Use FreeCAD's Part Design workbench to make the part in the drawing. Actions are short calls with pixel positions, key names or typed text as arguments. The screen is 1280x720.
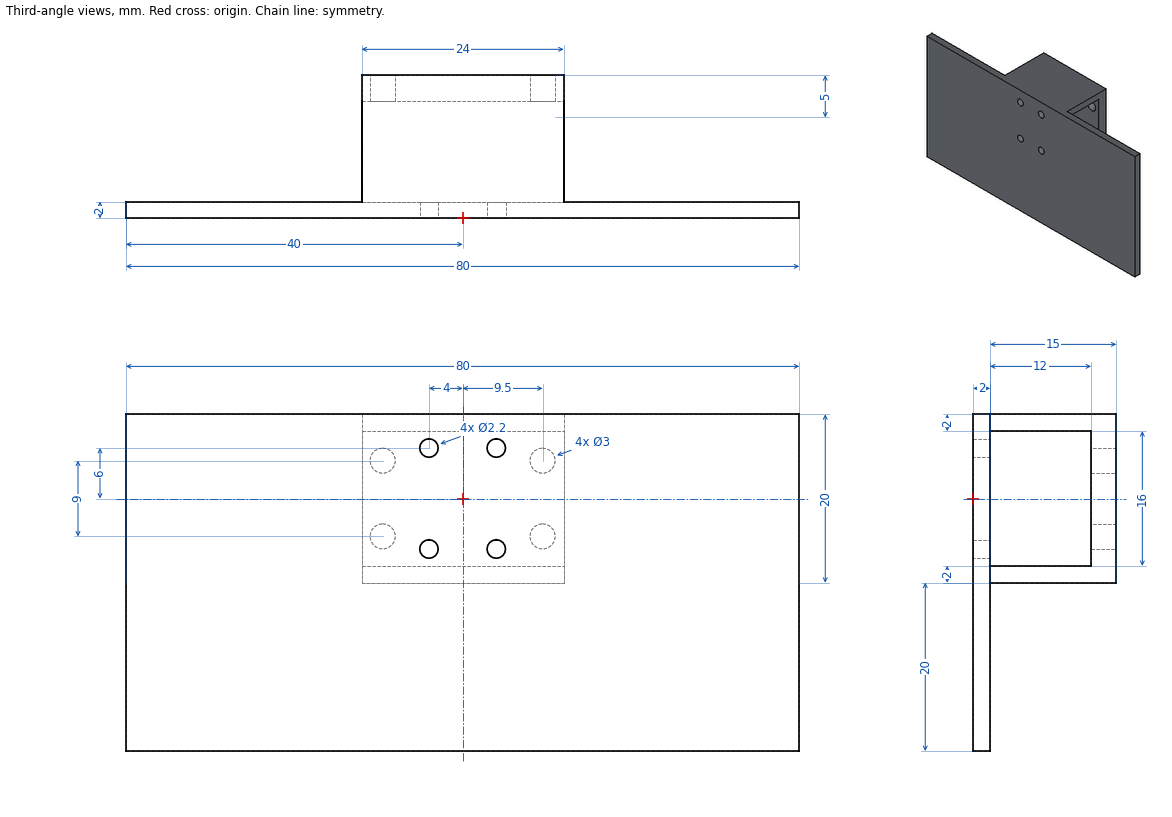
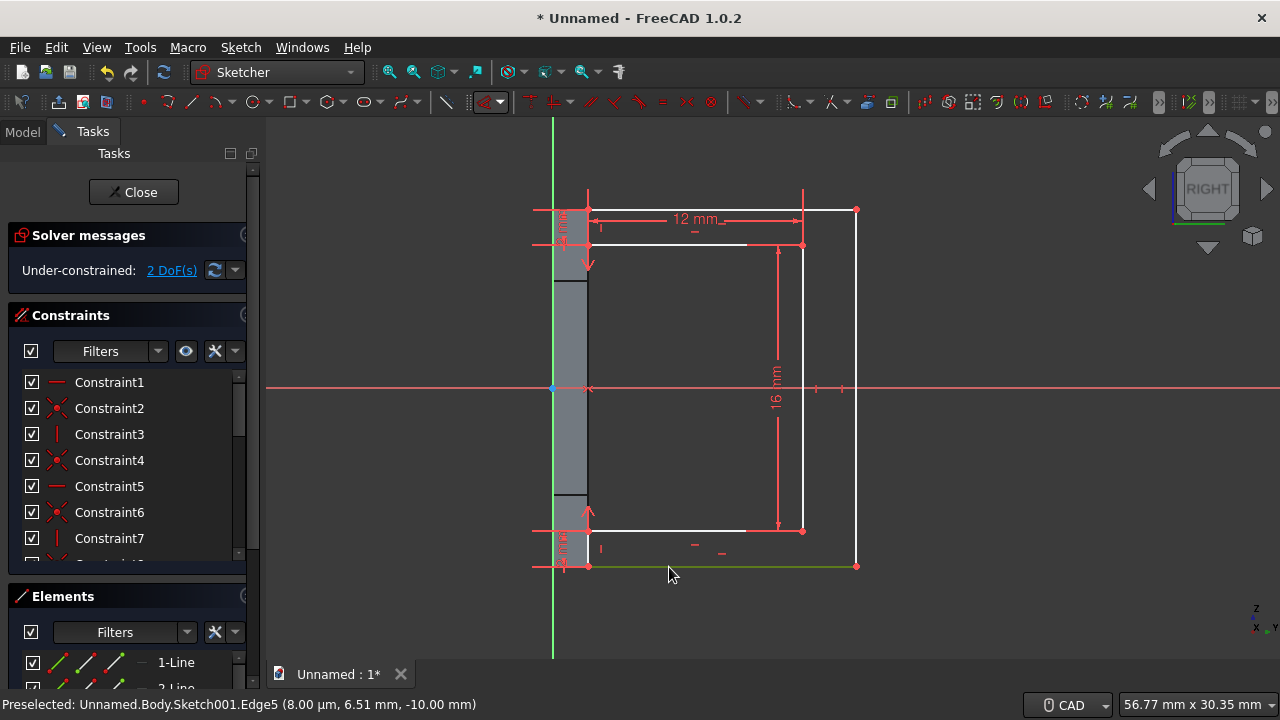
key(l)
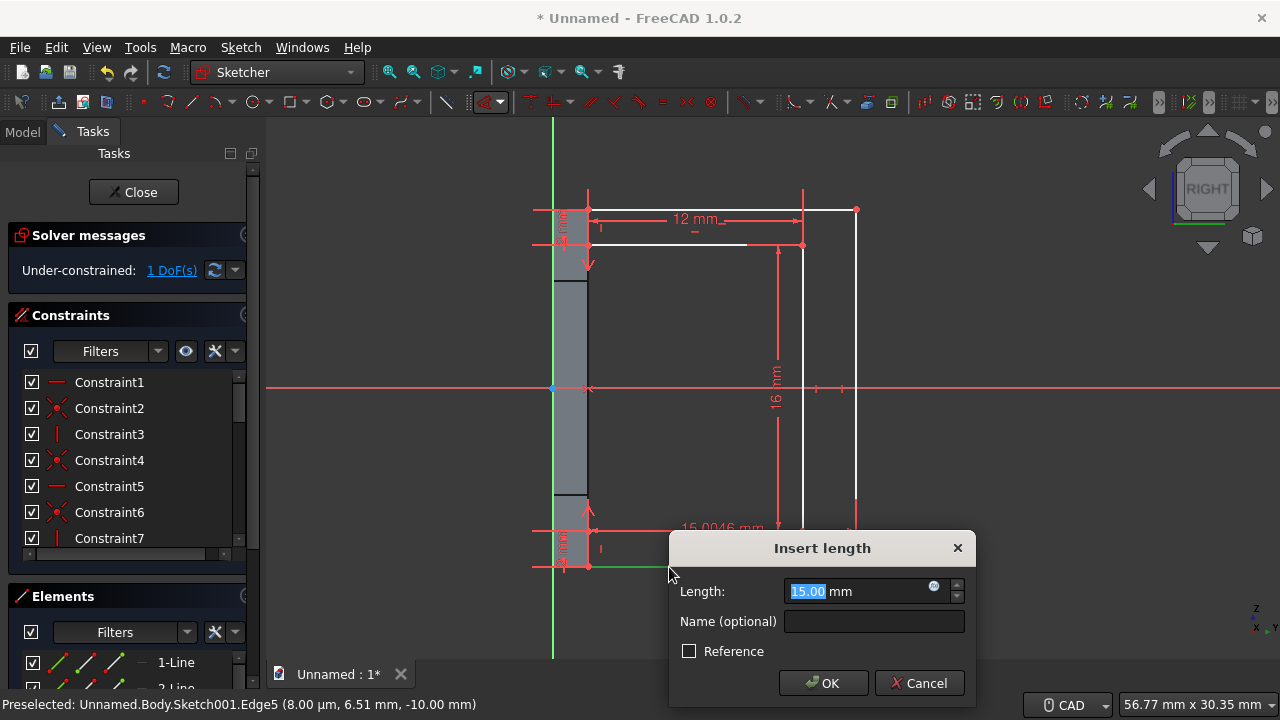
text(15)
key(Return)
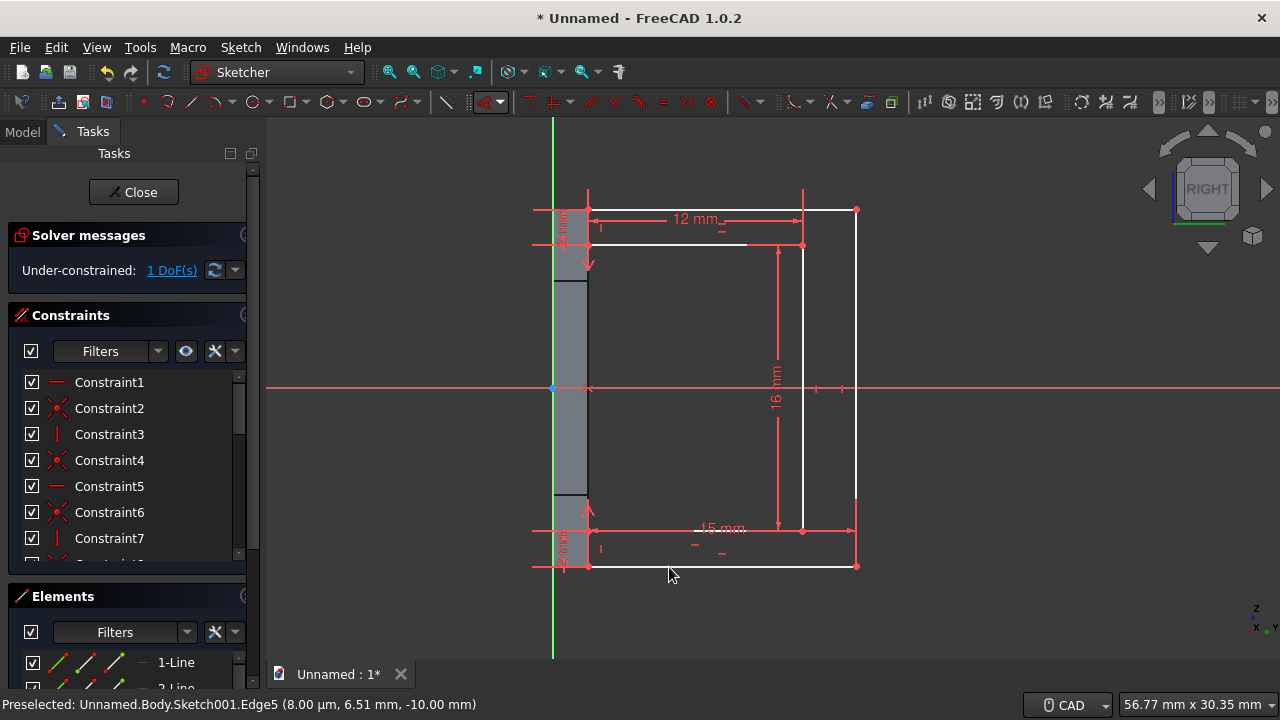
click(588, 245)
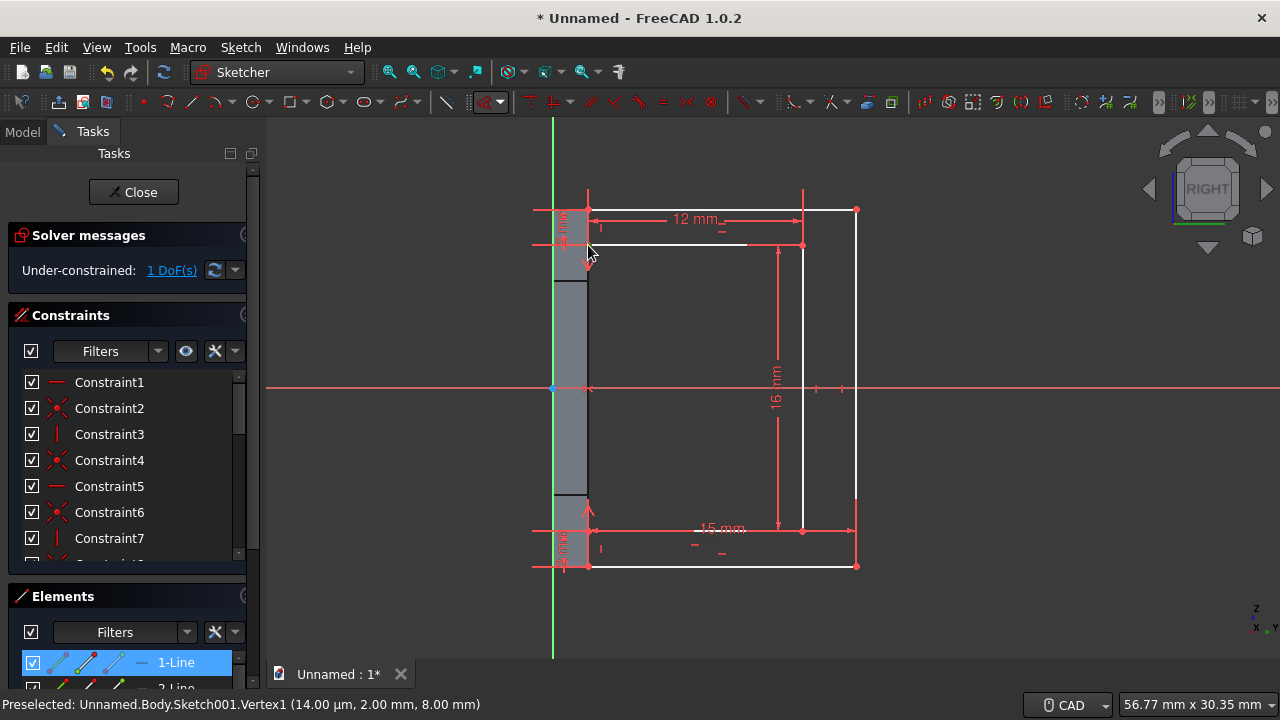
click(502, 102)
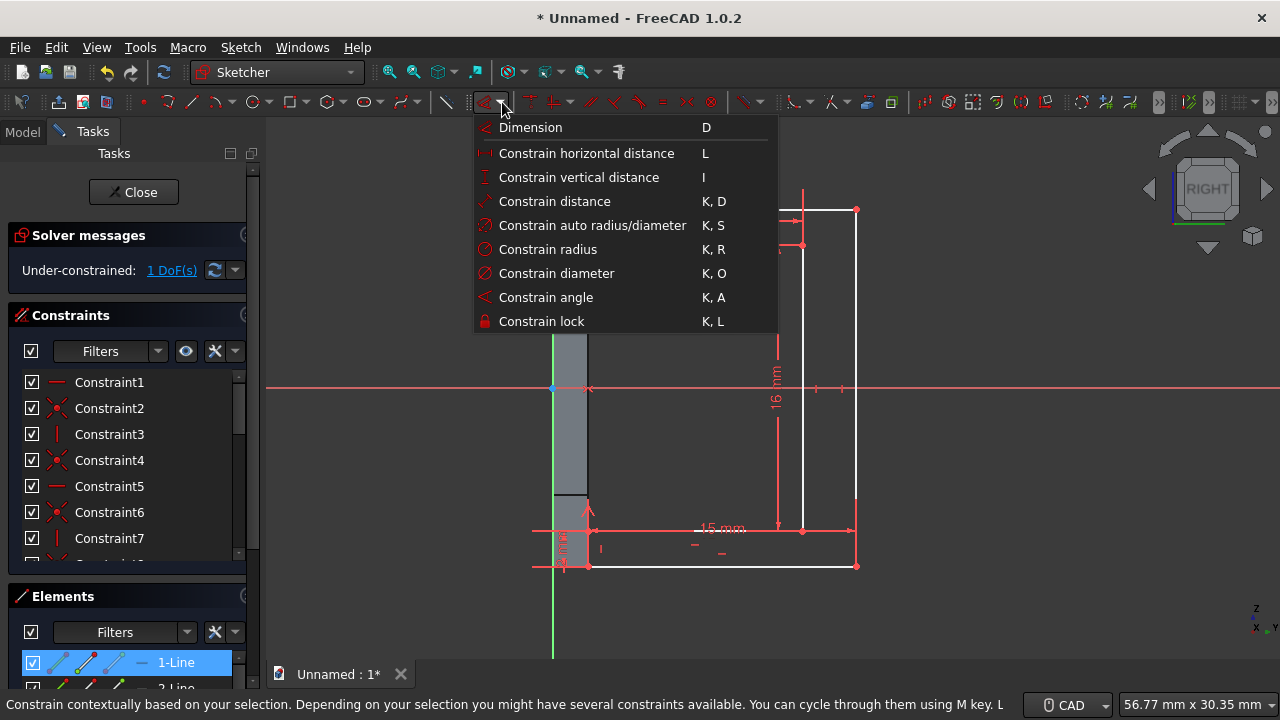
click(626, 153)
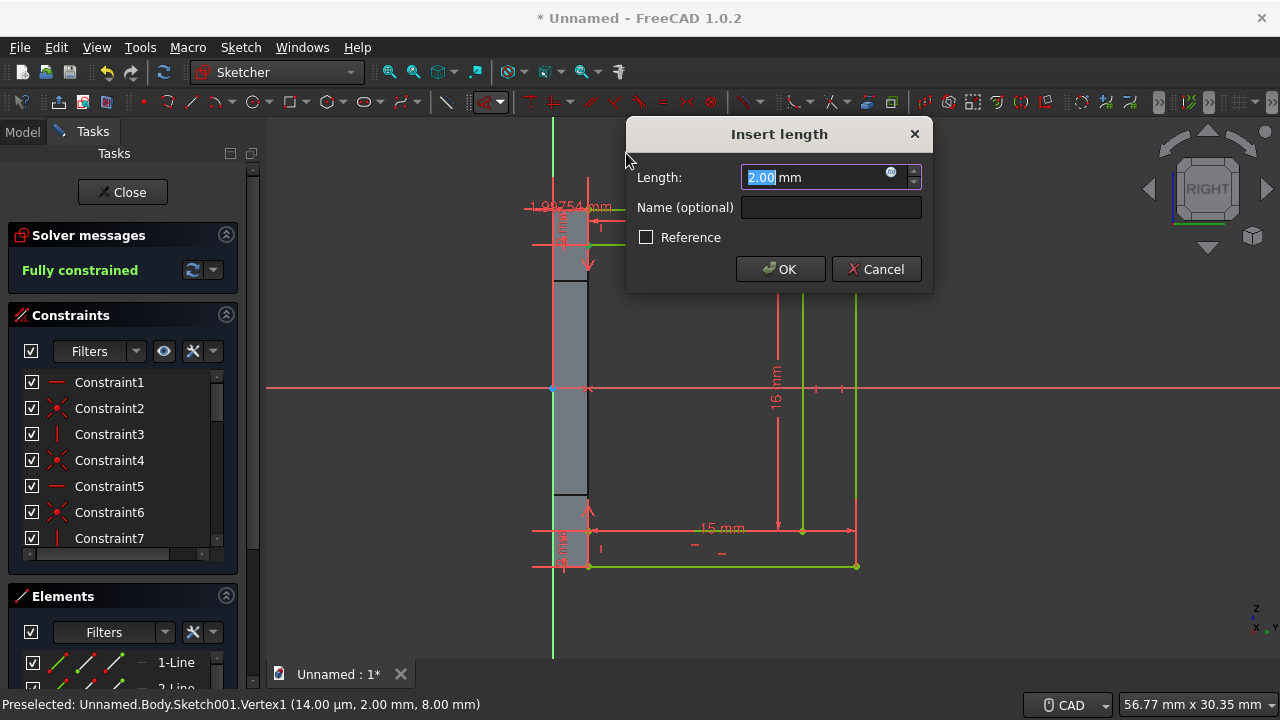
text(2)
key(Return)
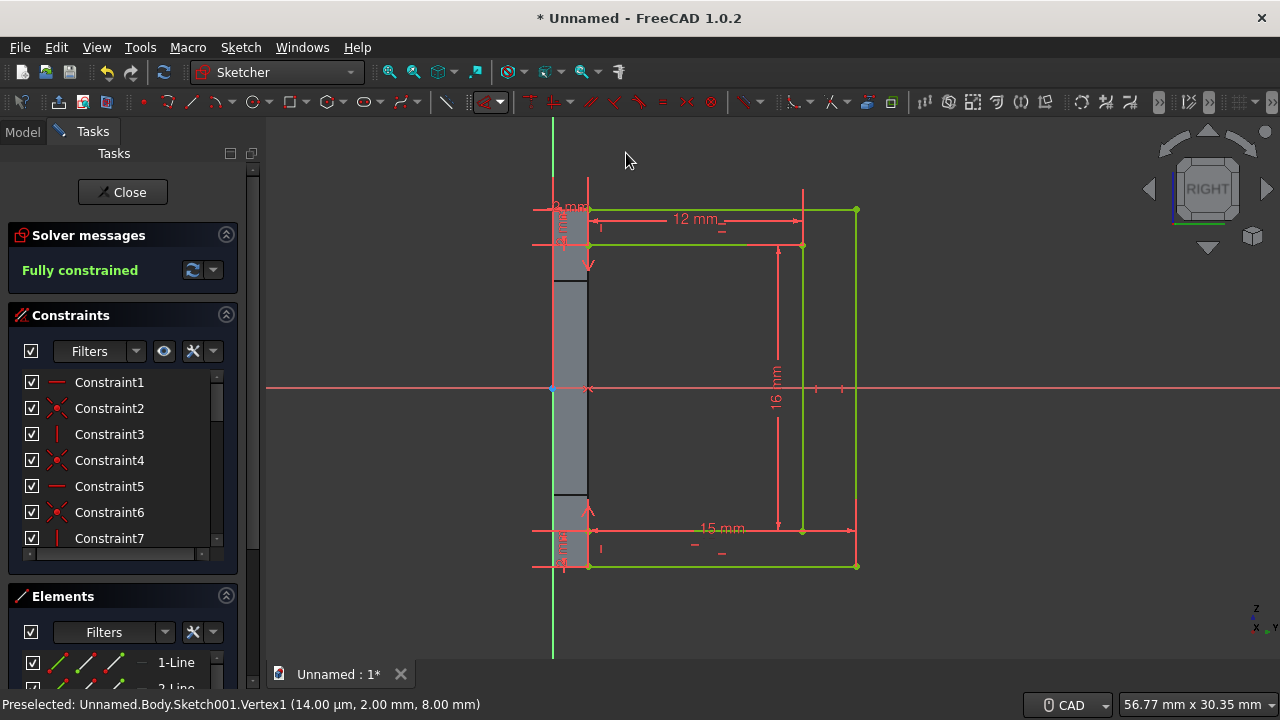
click(123, 192)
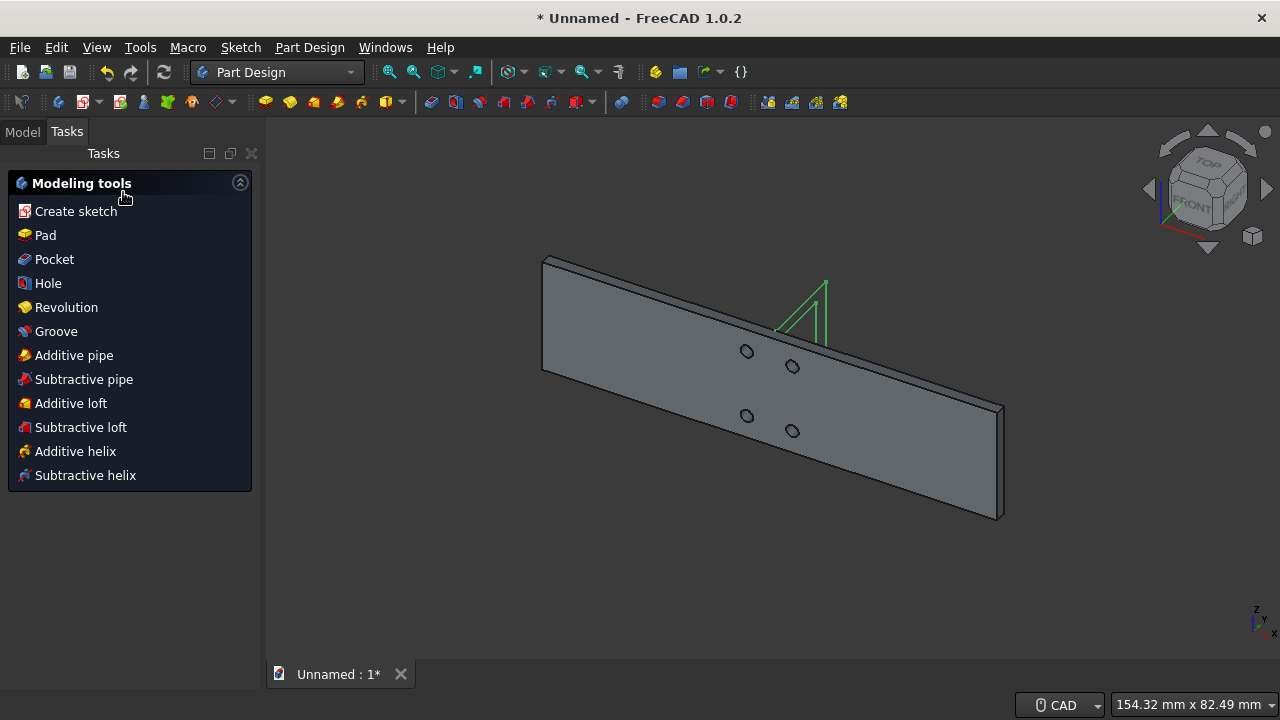
click(266, 102)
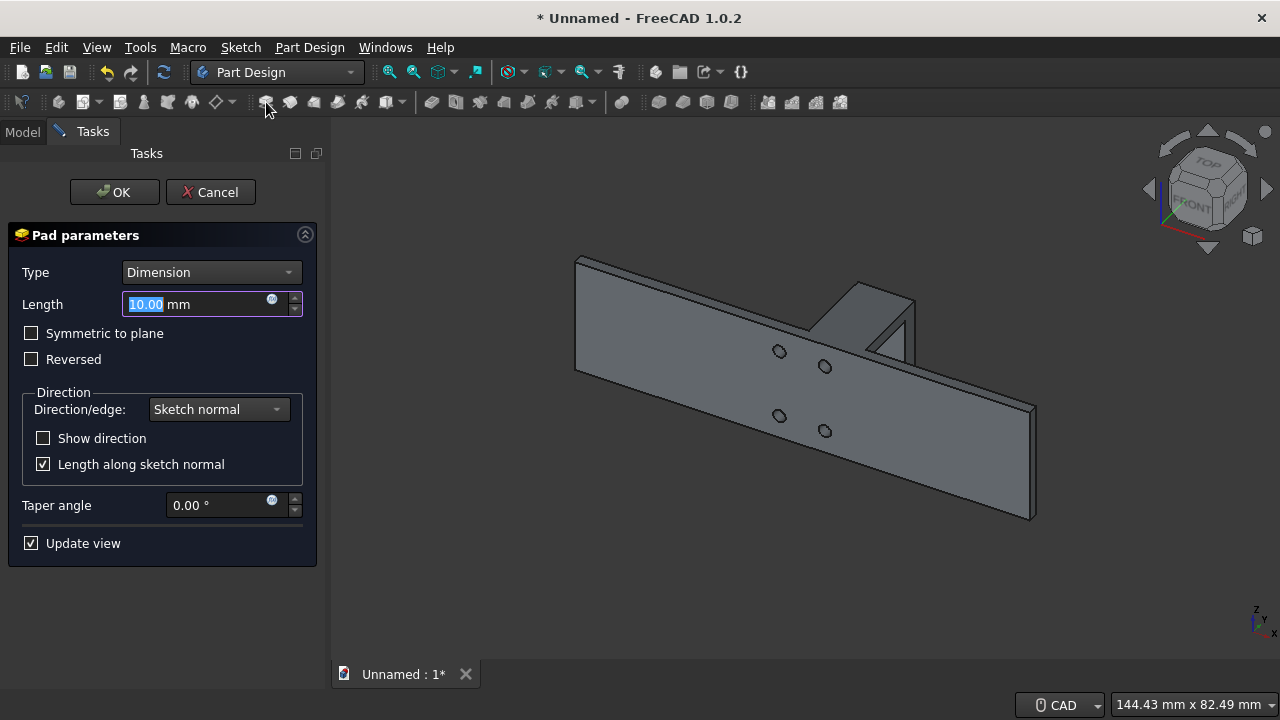
text(24)
key(Tab)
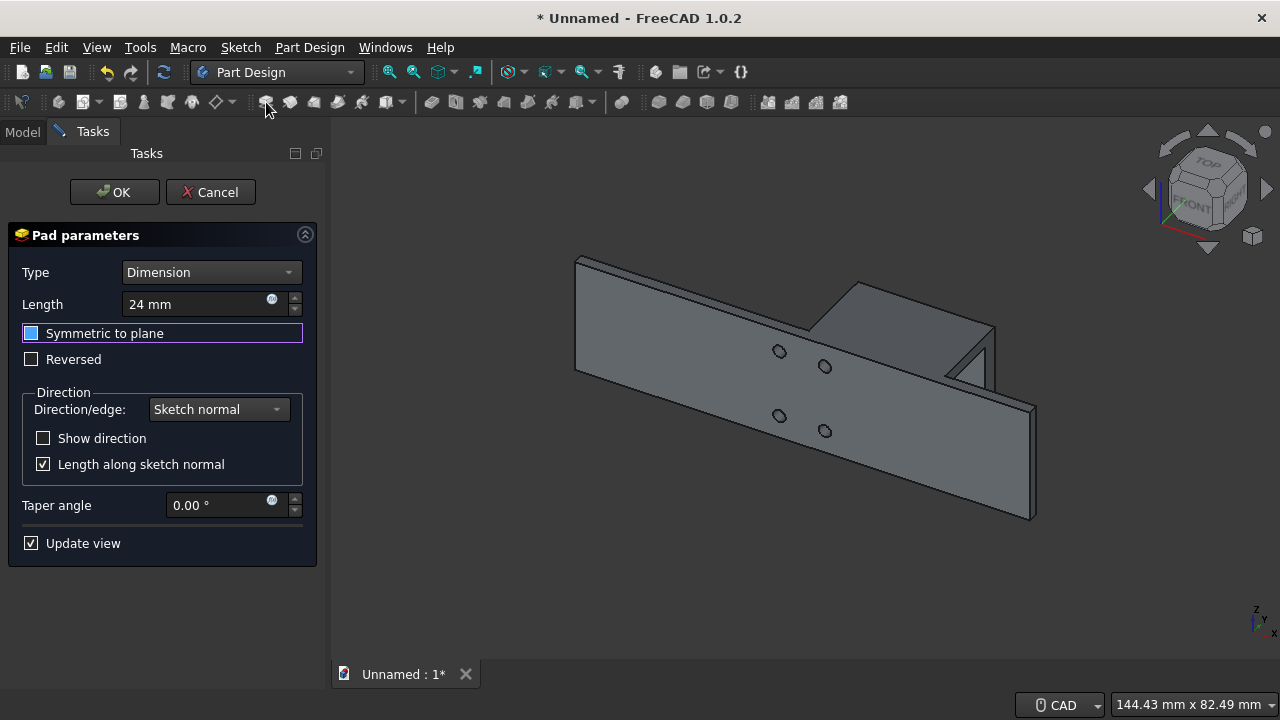
click(30, 333)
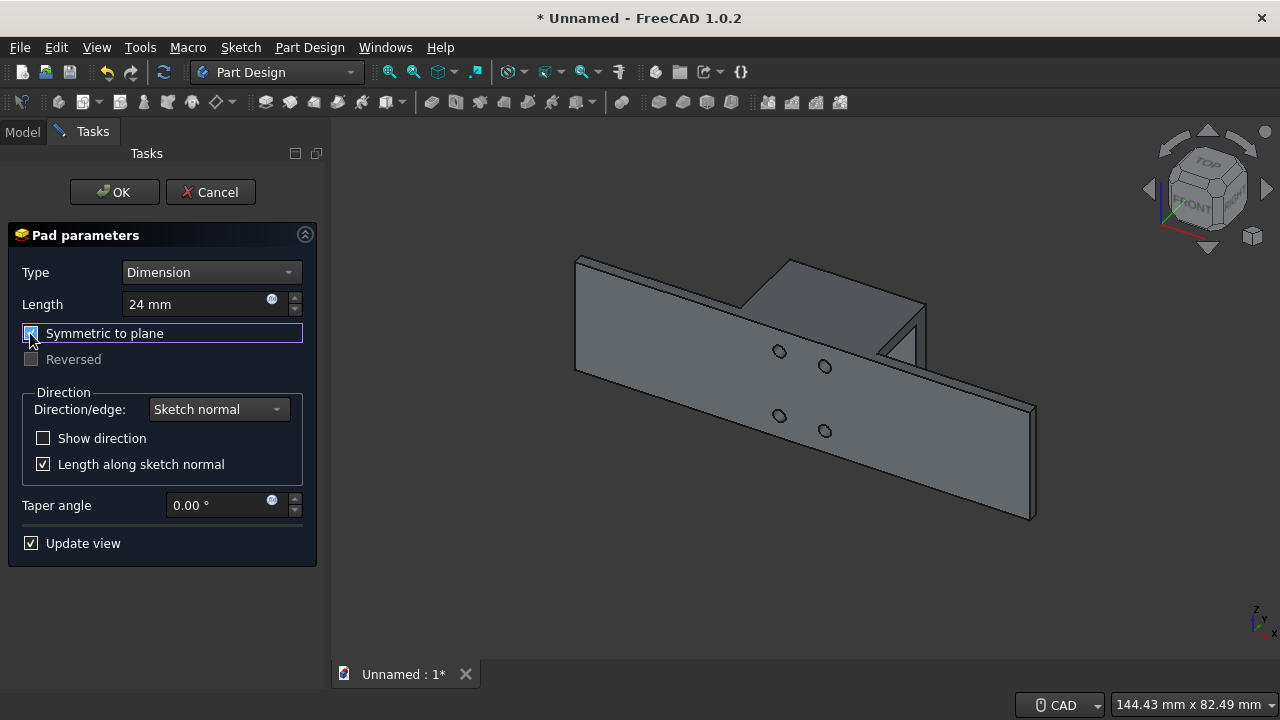
click(115, 192)